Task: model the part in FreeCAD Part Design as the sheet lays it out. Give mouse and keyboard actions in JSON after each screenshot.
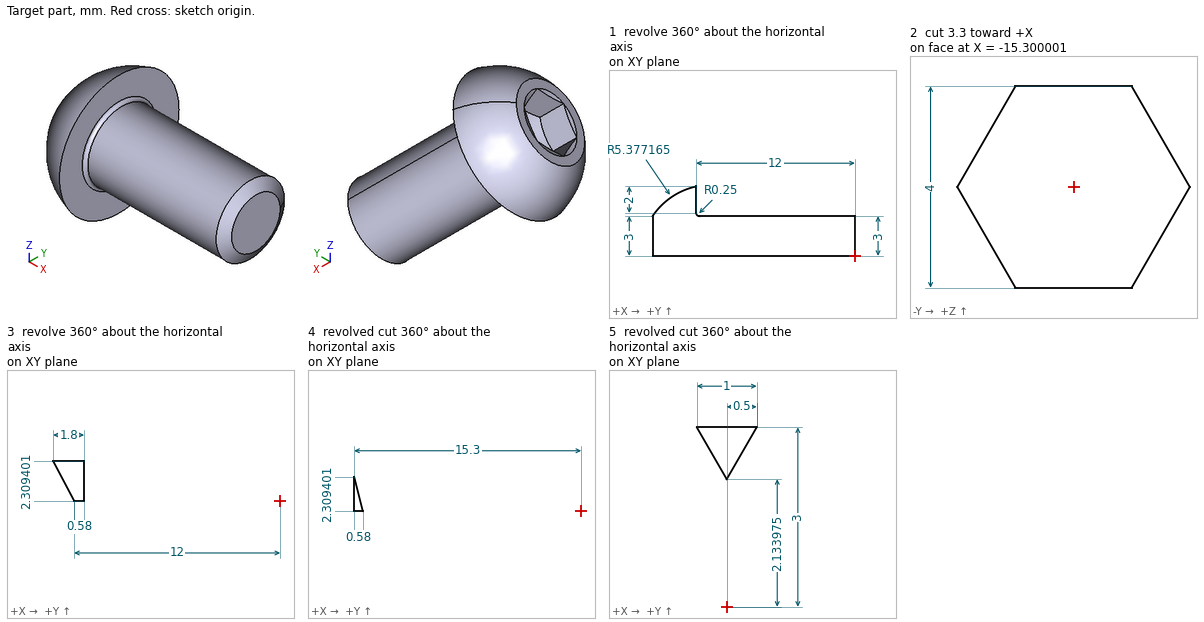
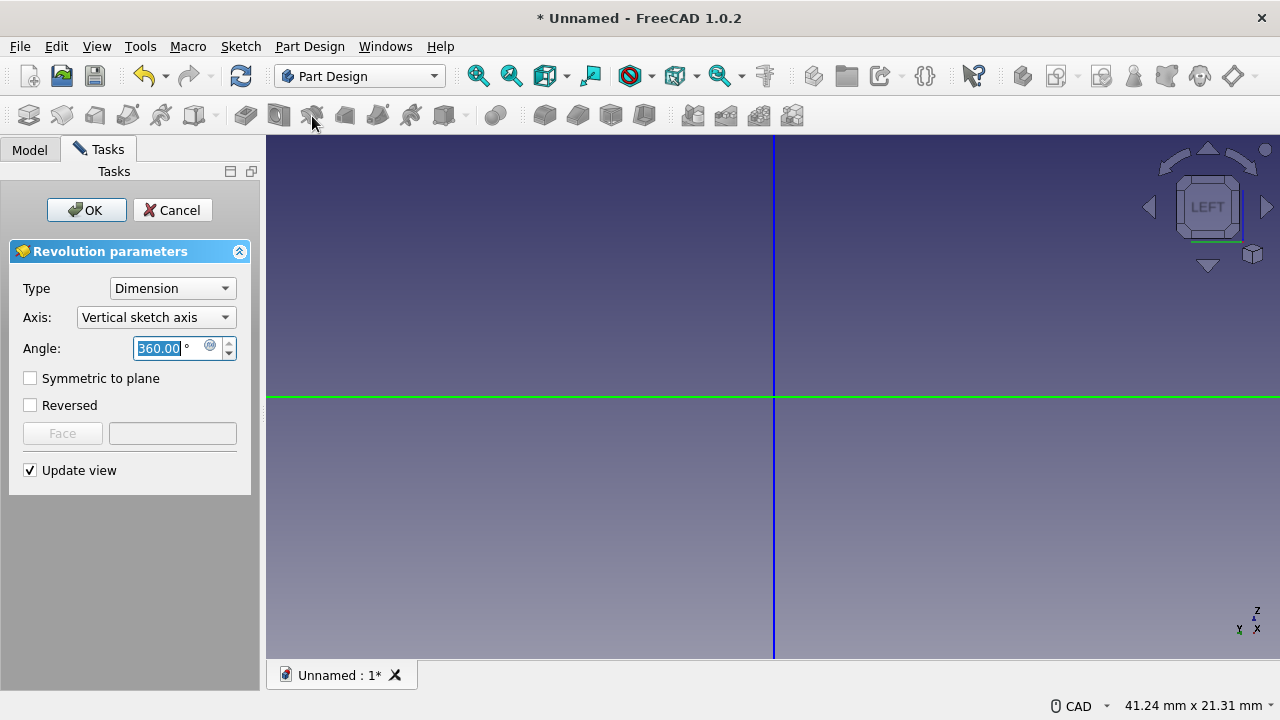
{"action": "left_click", "coordinate": [157, 318]}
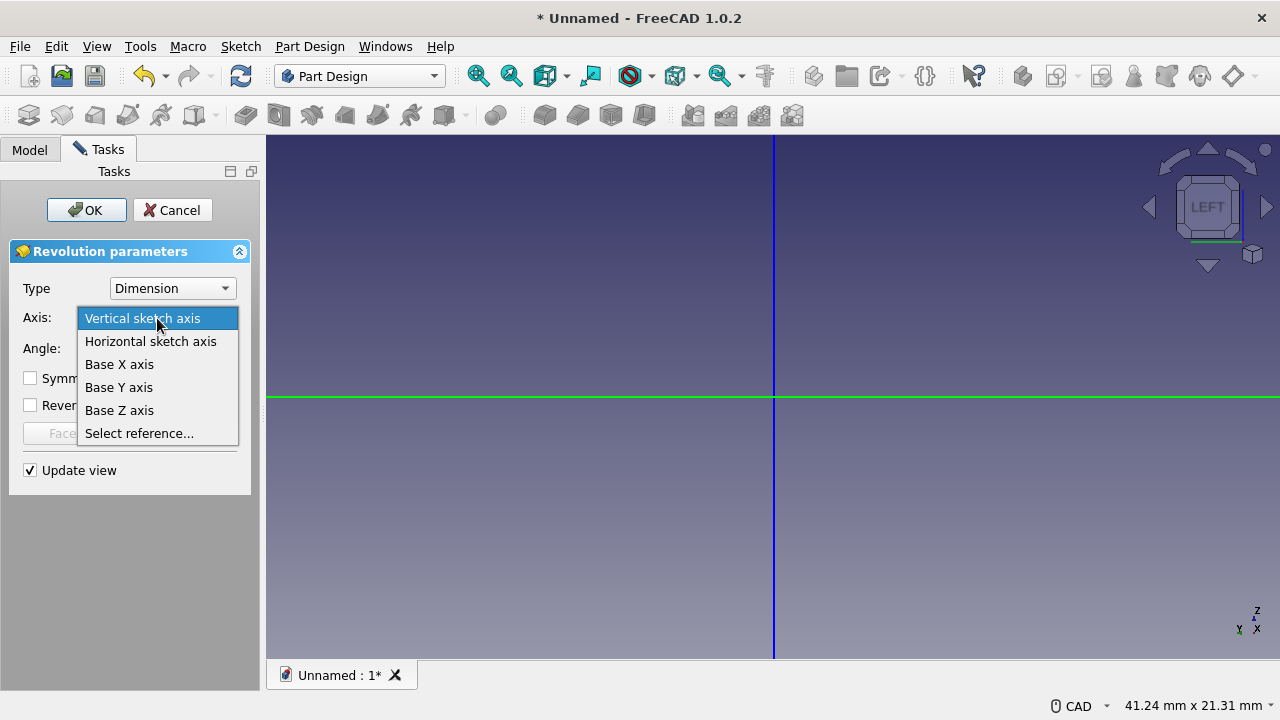
{"action": "left_click", "coordinate": [156, 342]}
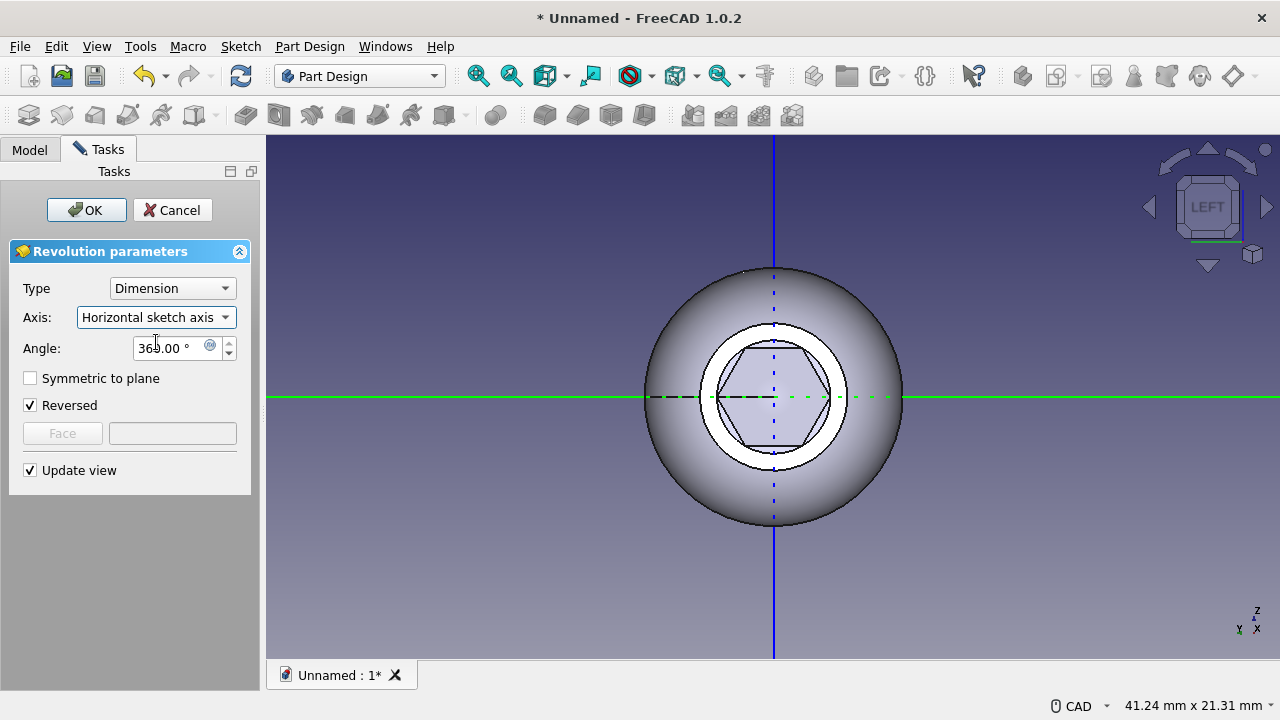
{"action": "left_click", "coordinate": [87, 210]}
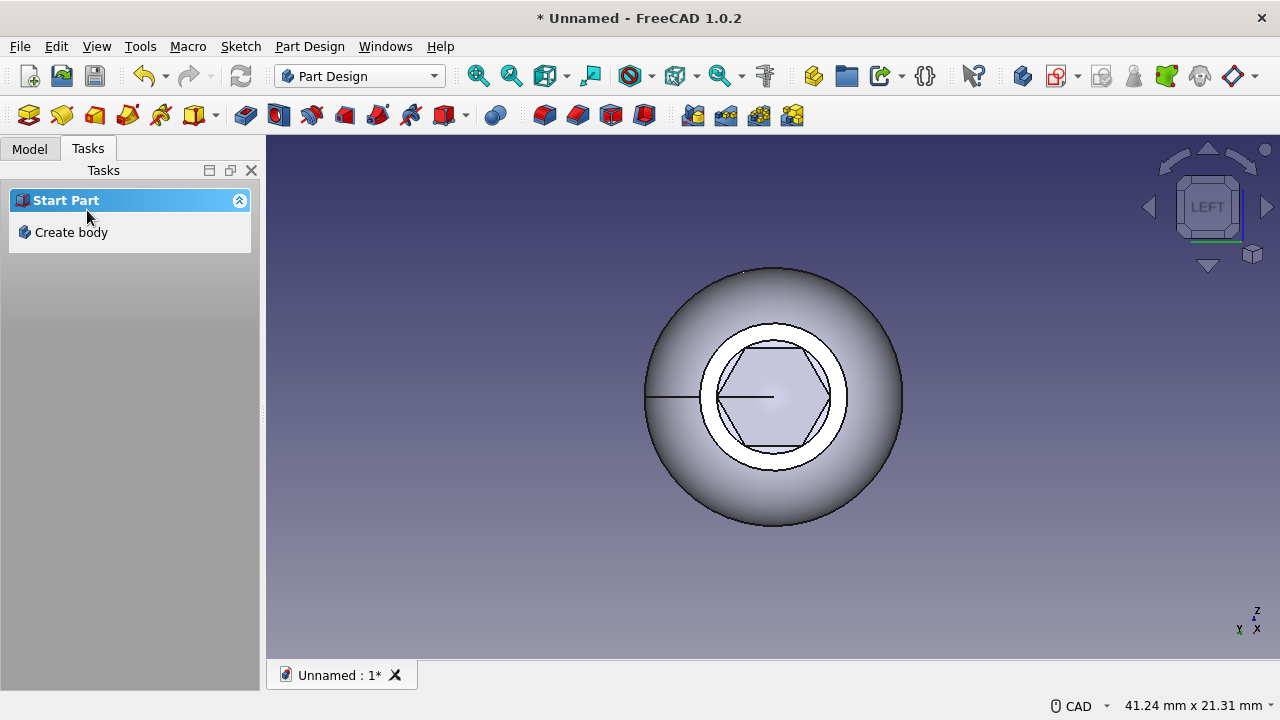
{"action": "key", "text": "0"}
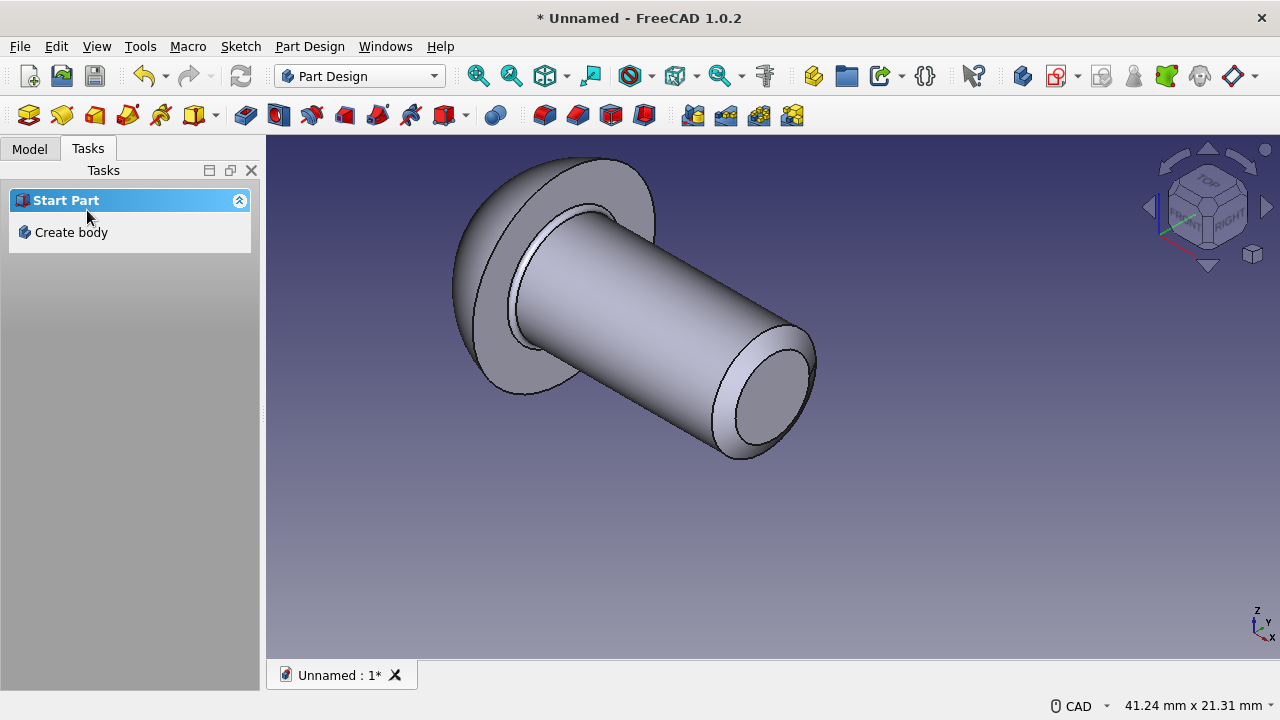
{"action": "left_click", "coordinate": [479, 76]}